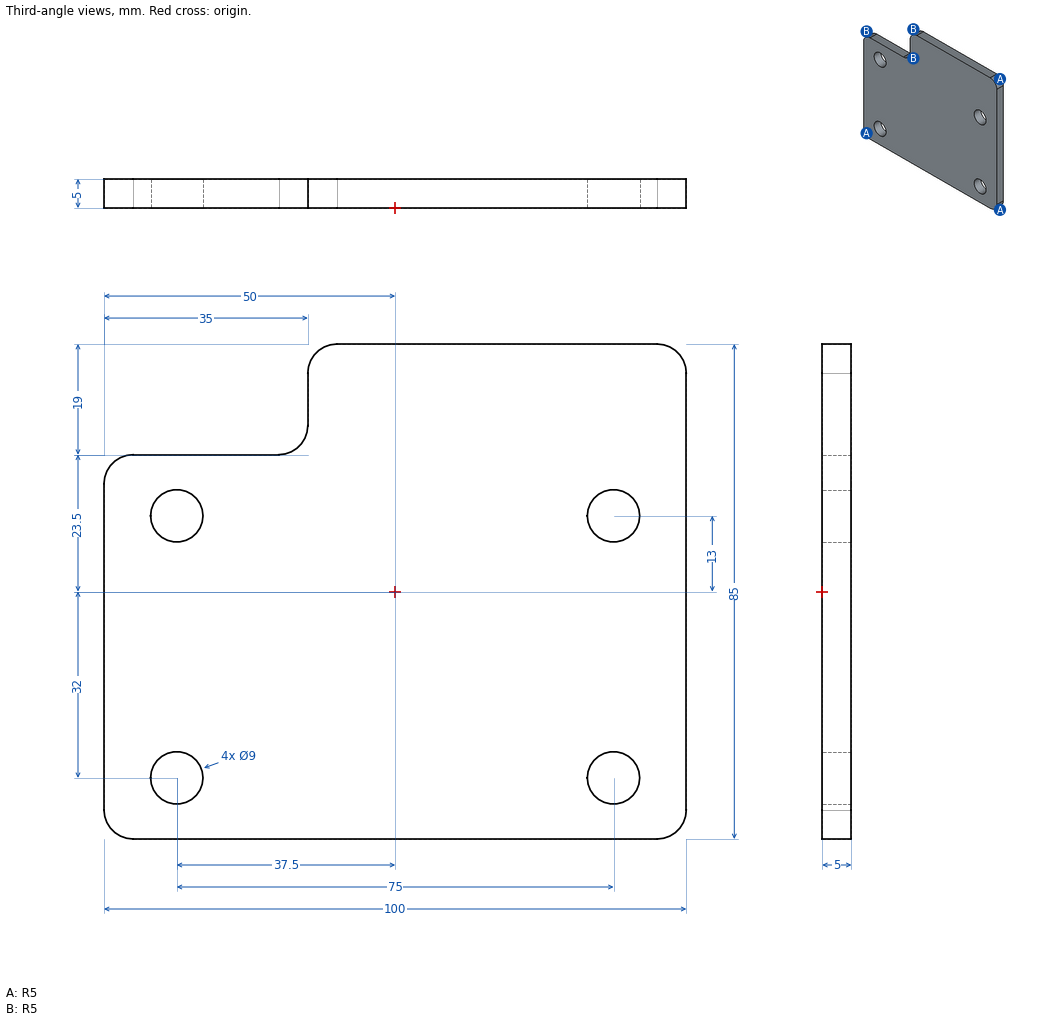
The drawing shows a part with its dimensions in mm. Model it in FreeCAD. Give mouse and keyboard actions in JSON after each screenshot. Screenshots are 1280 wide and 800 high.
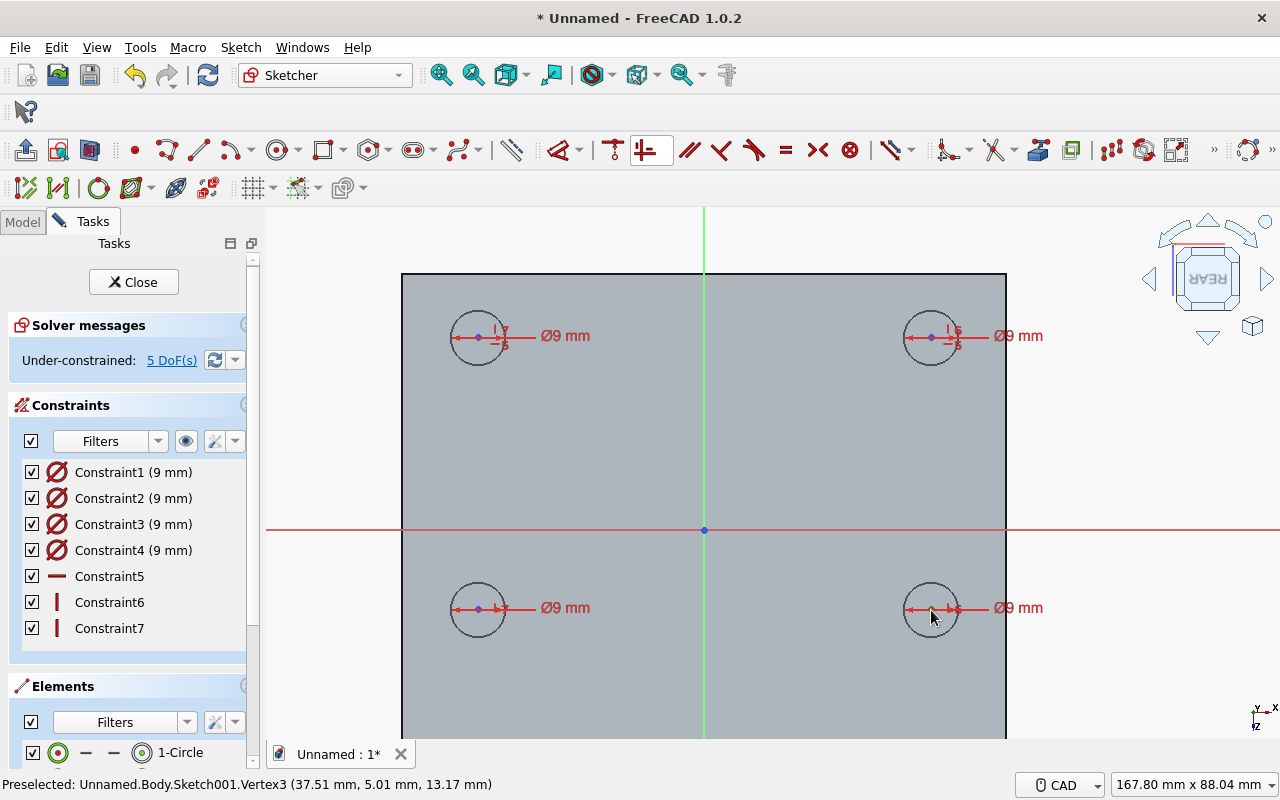
{"action": "left_click", "coordinate": [478, 610]}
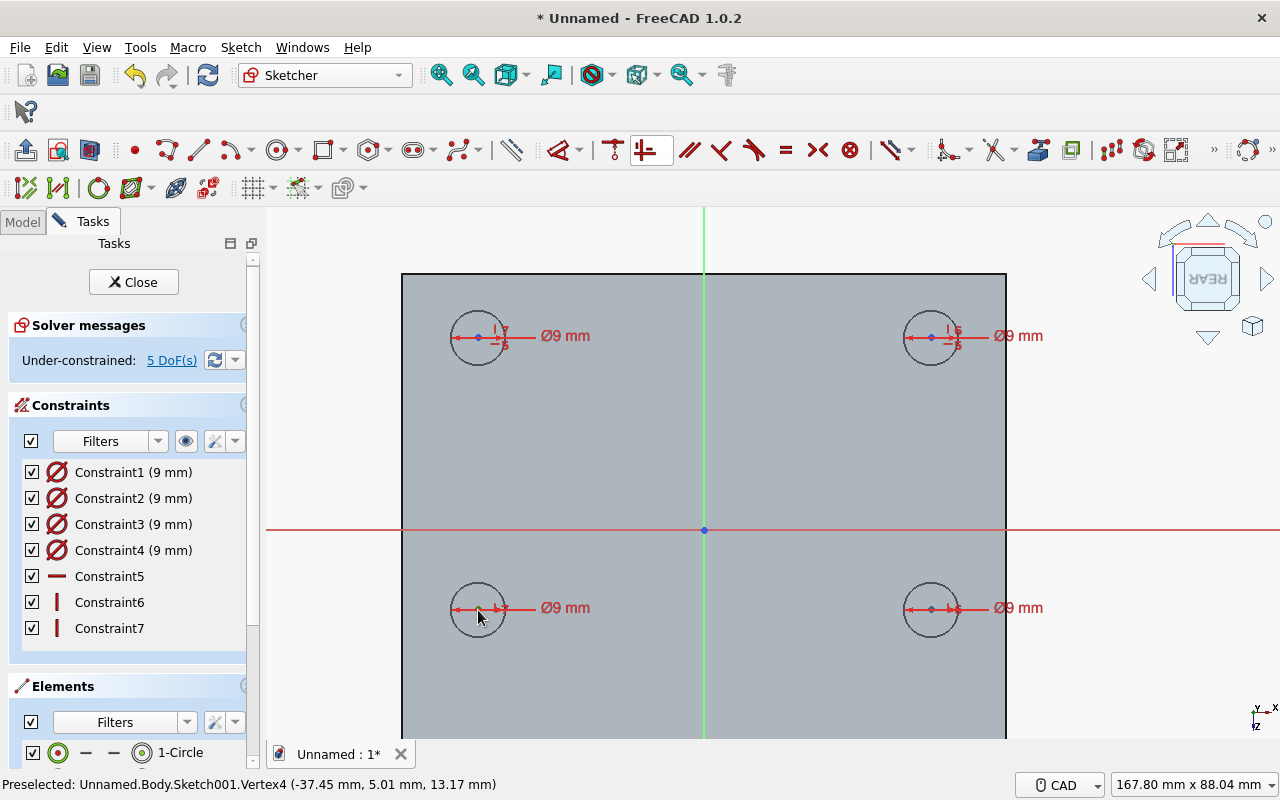
{"action": "left_click", "coordinate": [668, 150]}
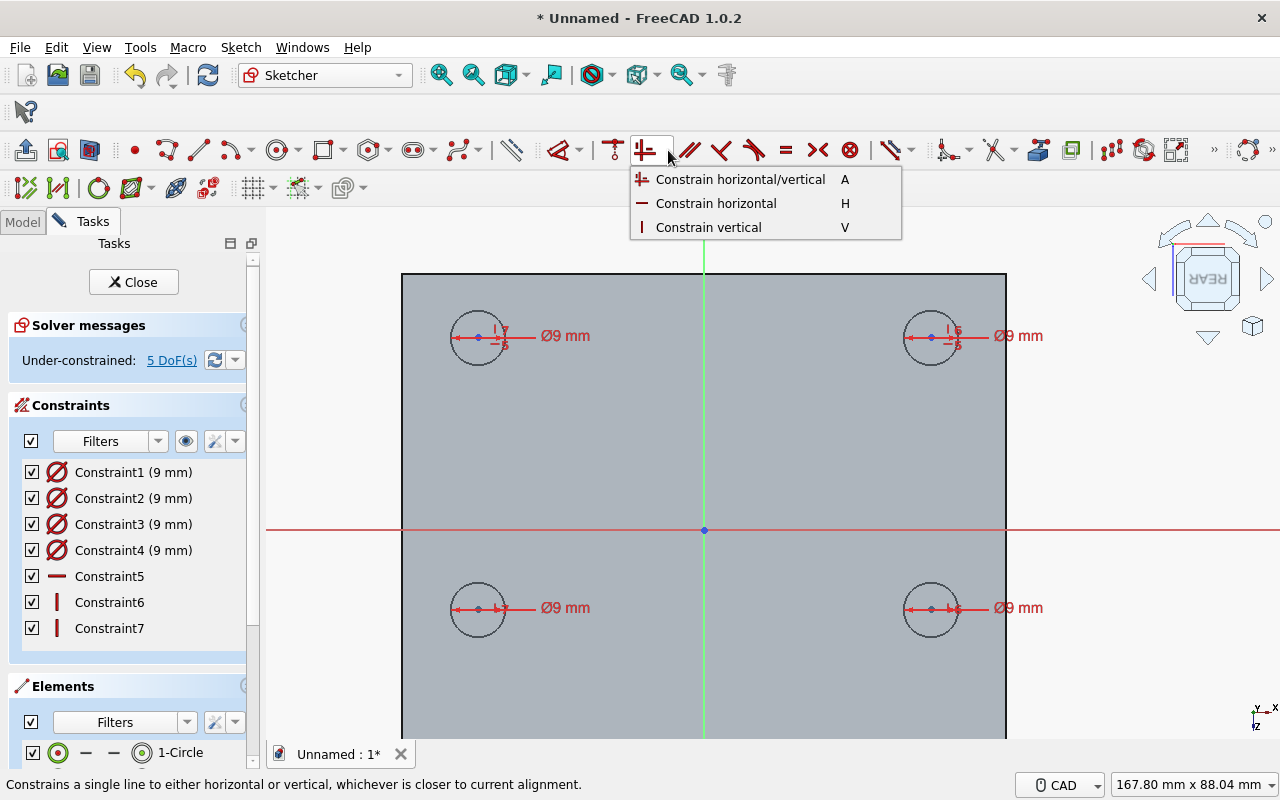
{"action": "left_click", "coordinate": [766, 203]}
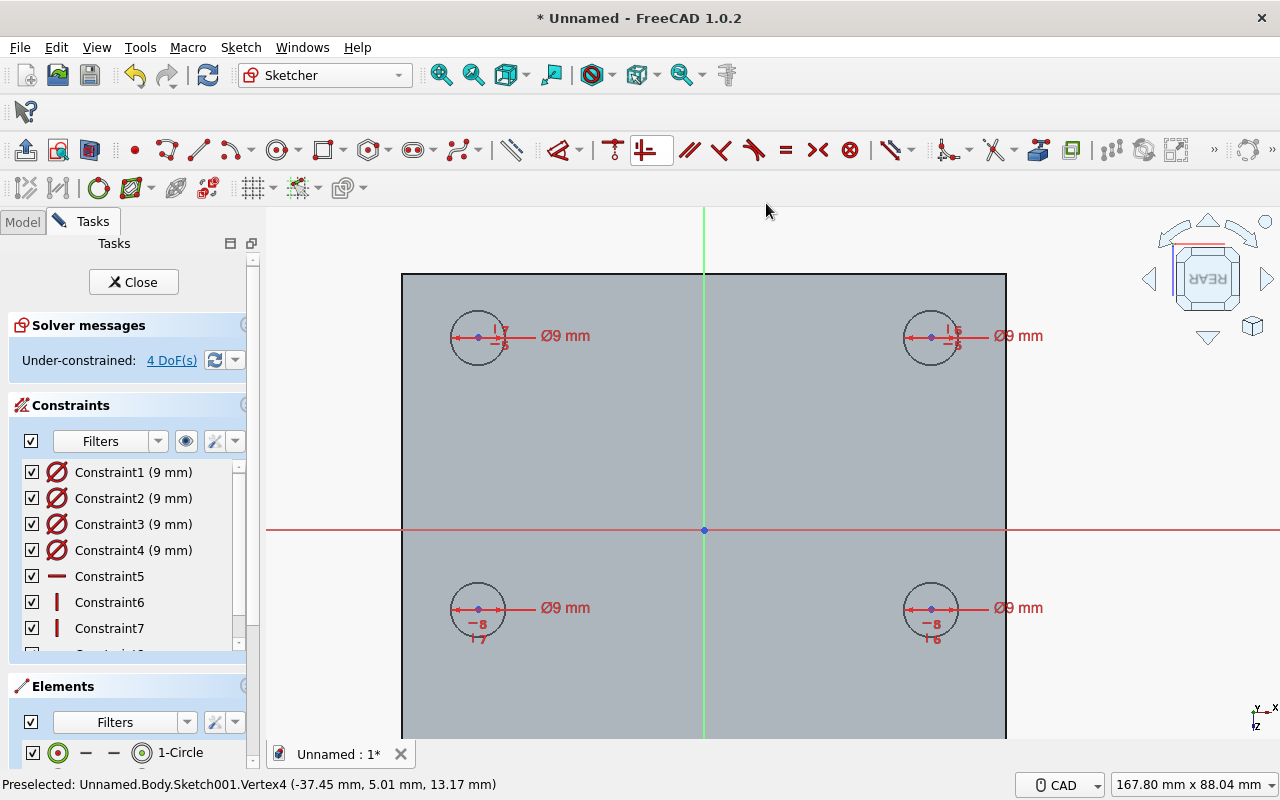
{"action": "left_click", "coordinate": [558, 150]}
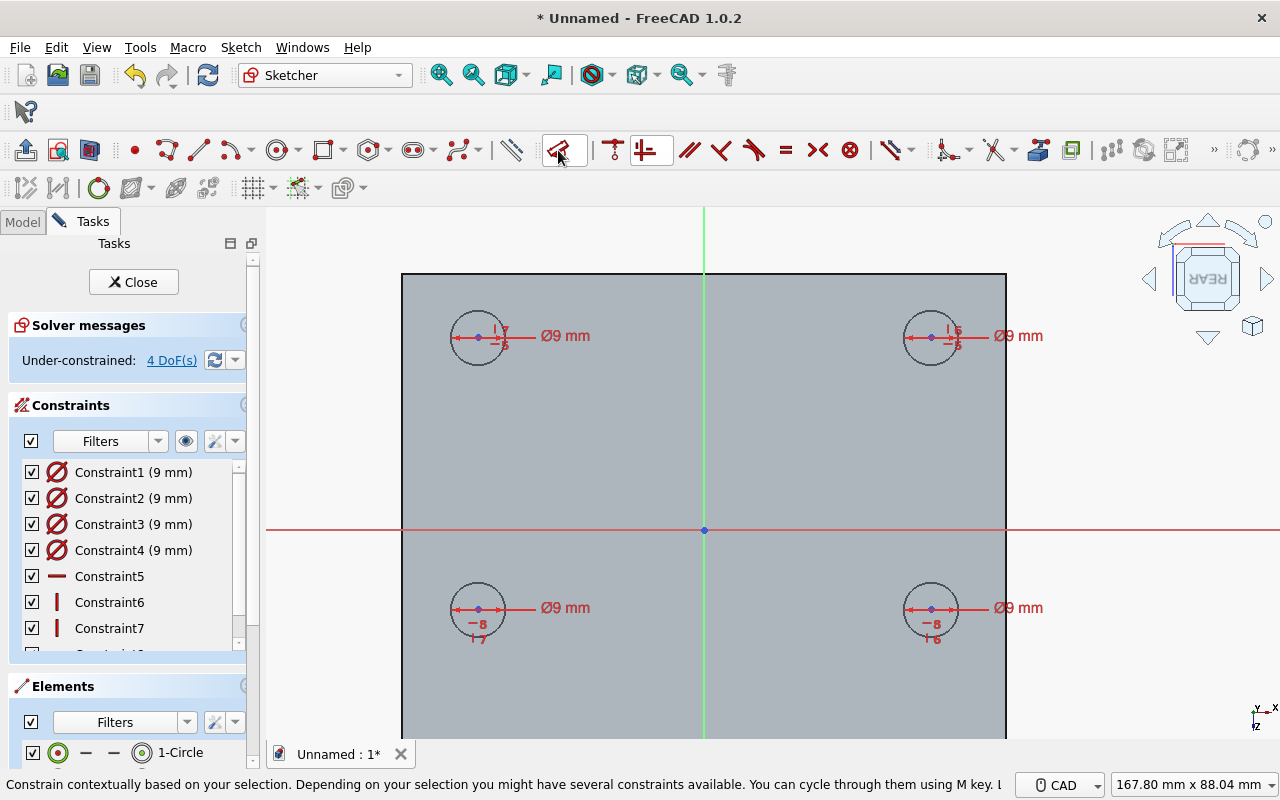
{"action": "left_click", "coordinate": [478, 338]}
{"action": "left_click", "coordinate": [444, 434]}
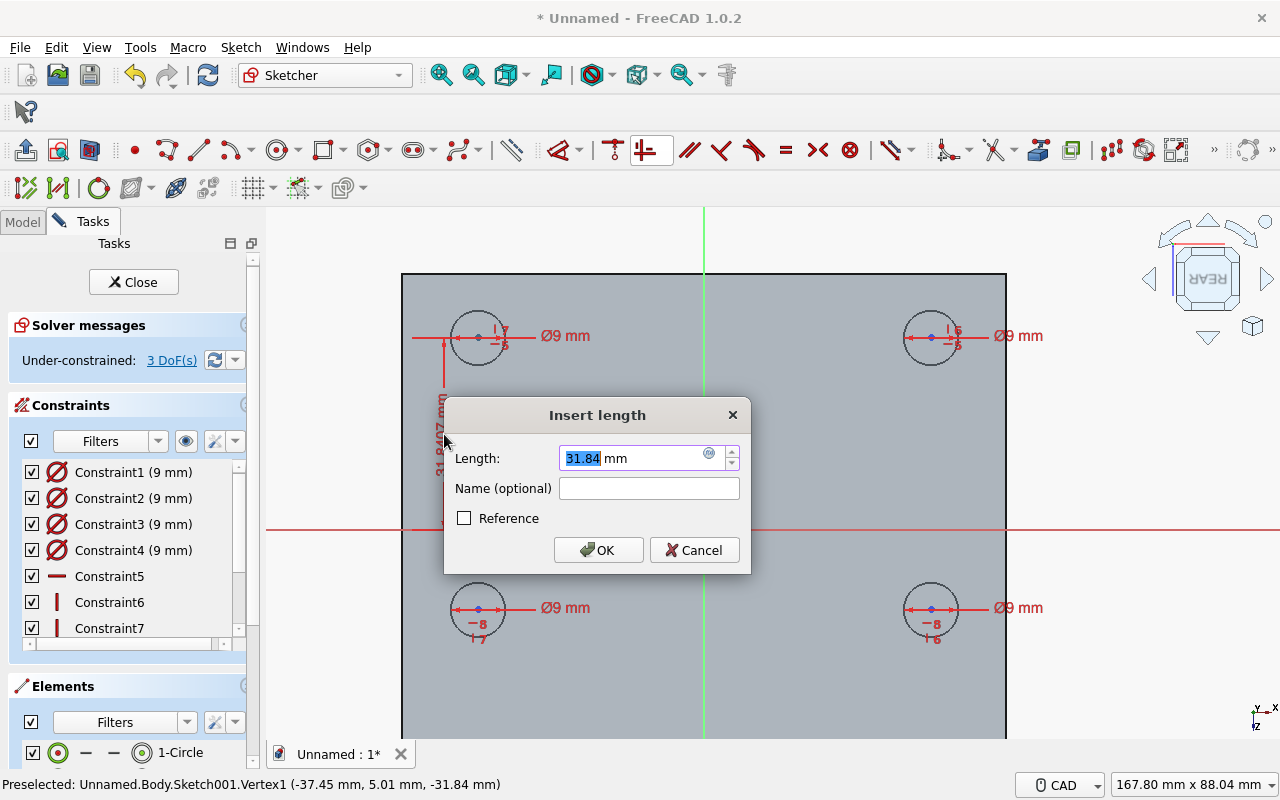
{"action": "type", "text": "32"}
{"action": "key", "text": "Return"}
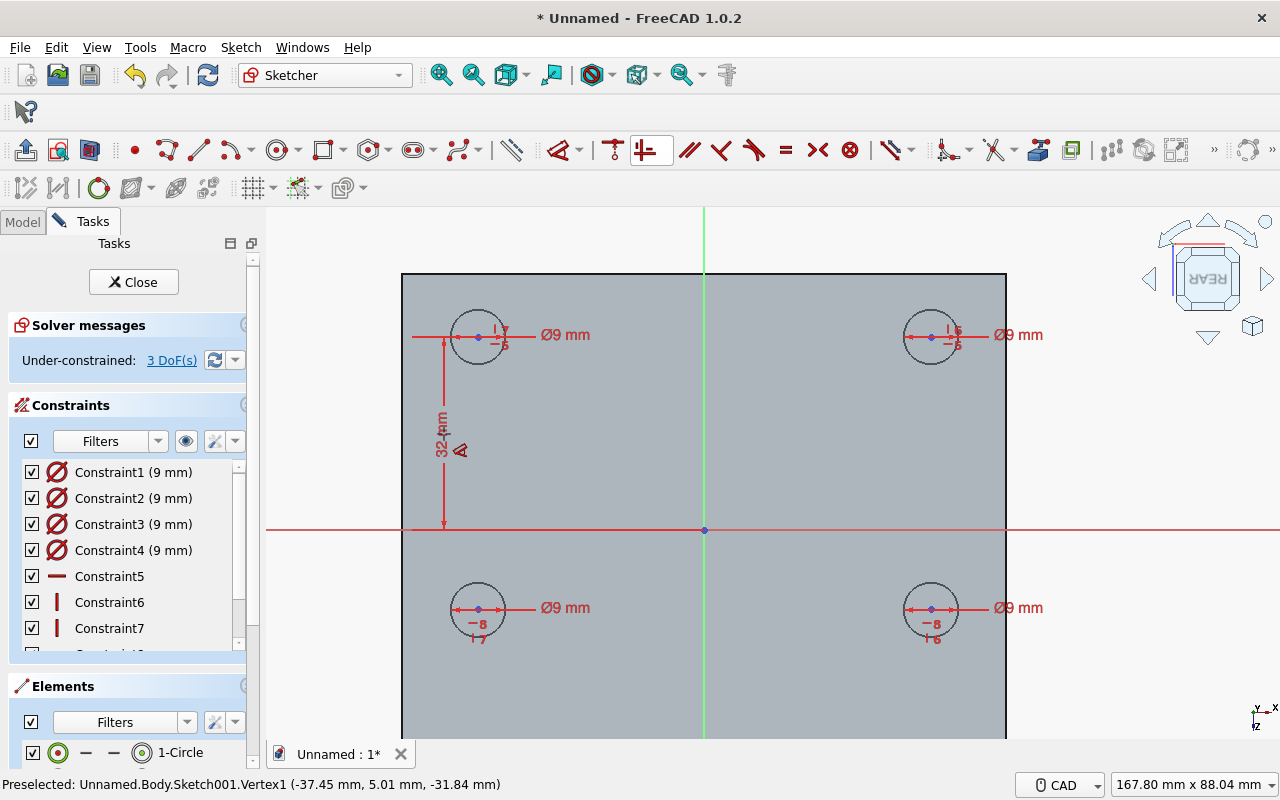
{"action": "left_click", "coordinate": [931, 610]}
{"action": "left_click", "coordinate": [965, 570]}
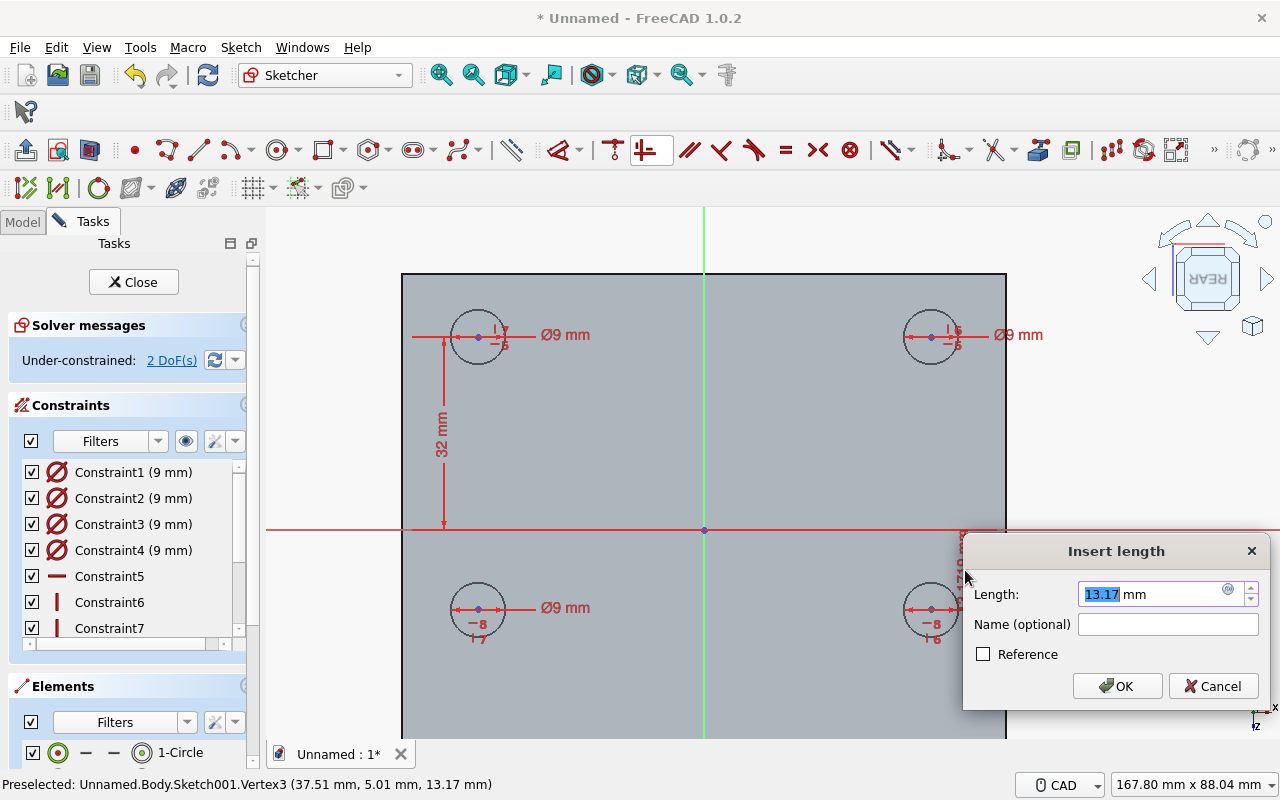
{"action": "type", "text": "13"}
{"action": "key", "text": "Return"}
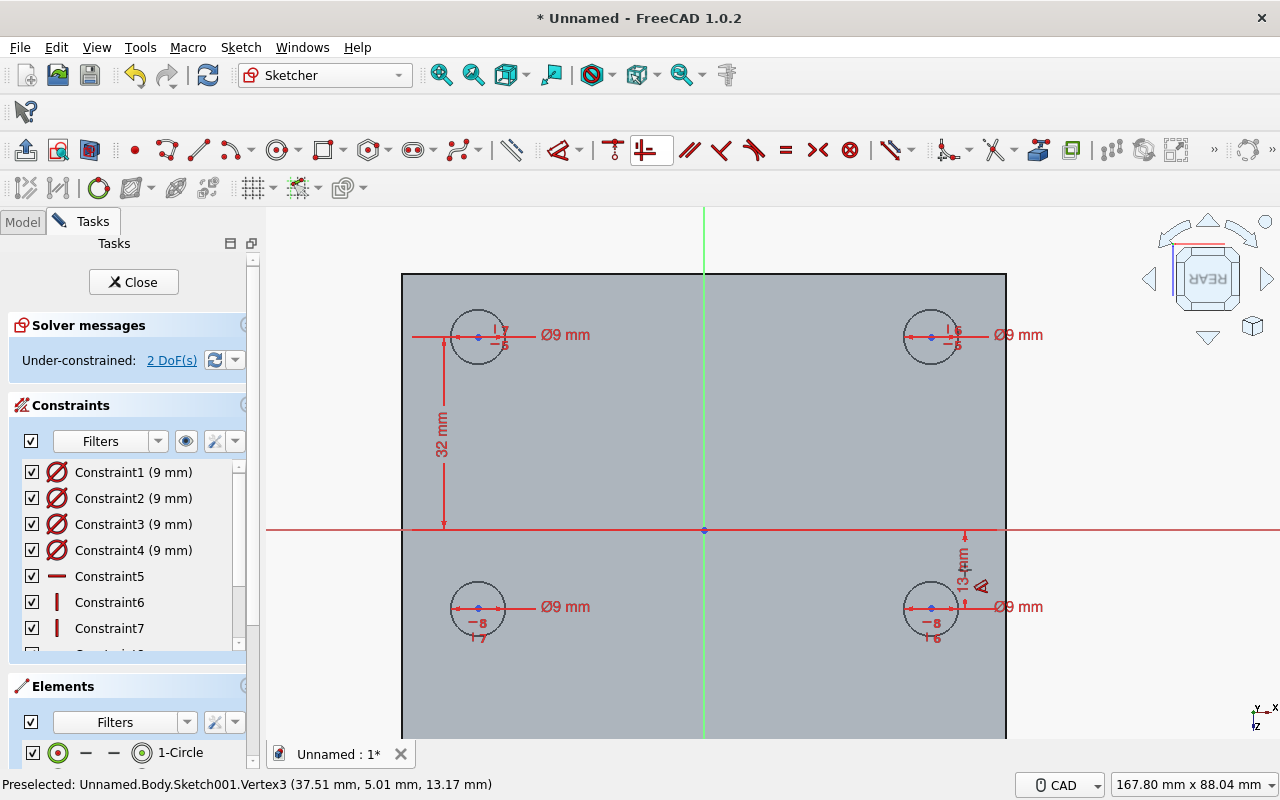
{"action": "left_click", "coordinate": [478, 337]}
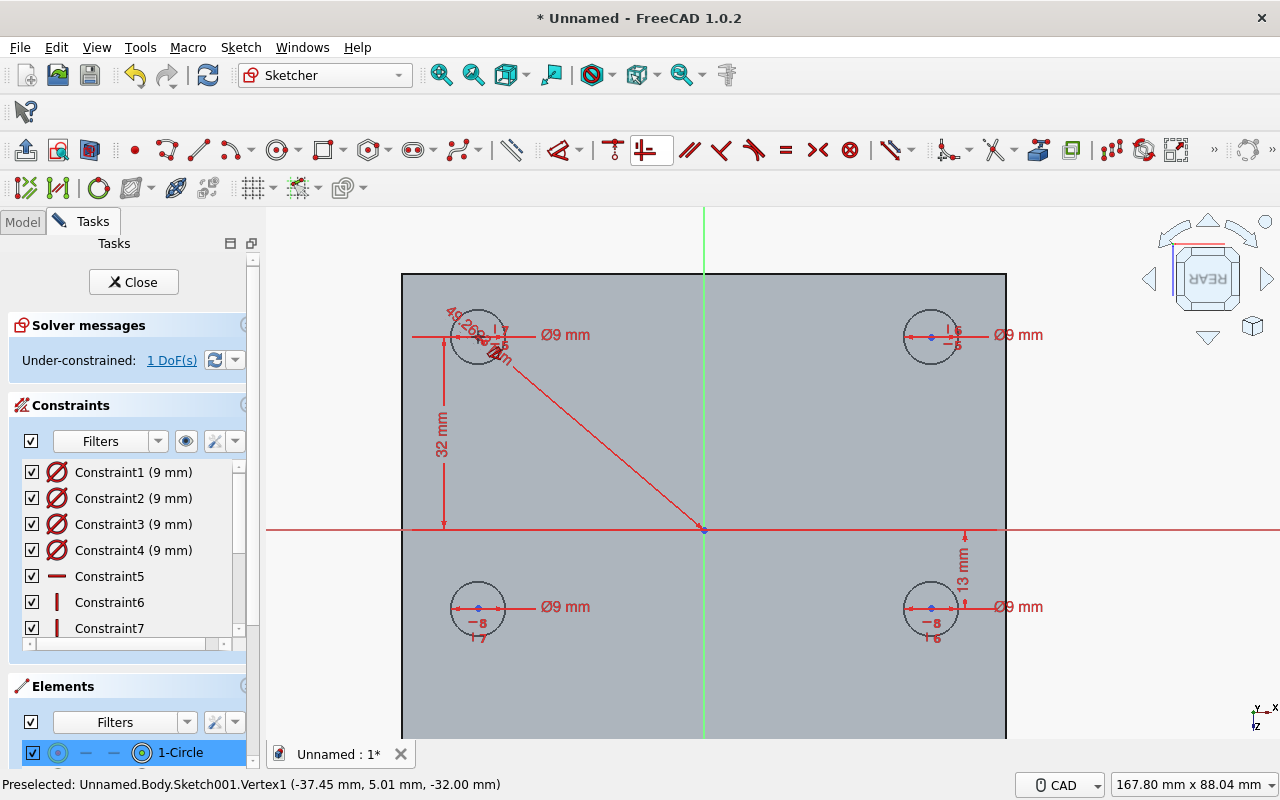
{"action": "left_click", "coordinate": [931, 337]}
{"action": "left_click", "coordinate": [600, 303]}